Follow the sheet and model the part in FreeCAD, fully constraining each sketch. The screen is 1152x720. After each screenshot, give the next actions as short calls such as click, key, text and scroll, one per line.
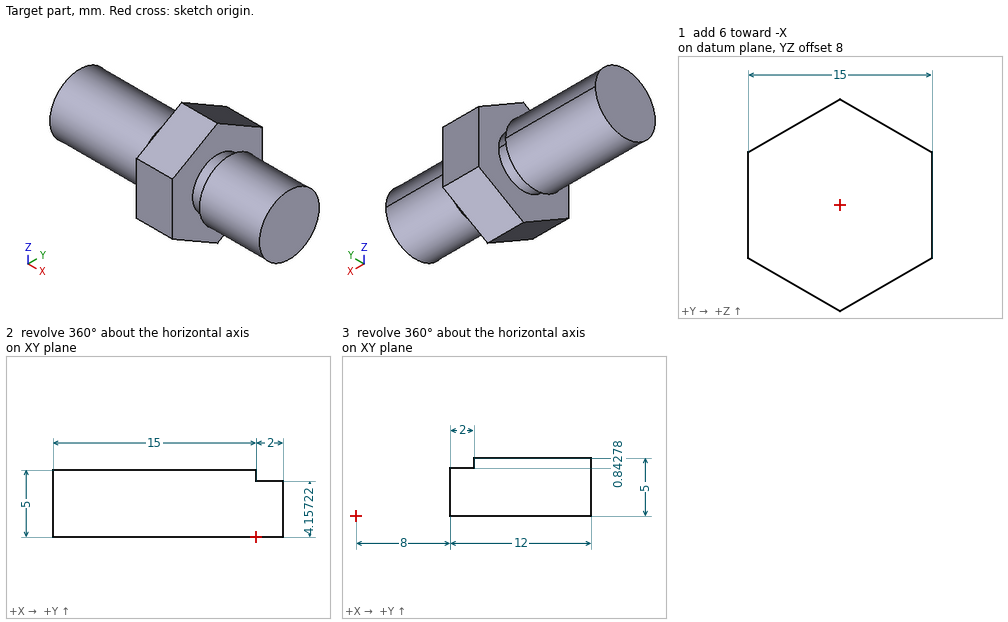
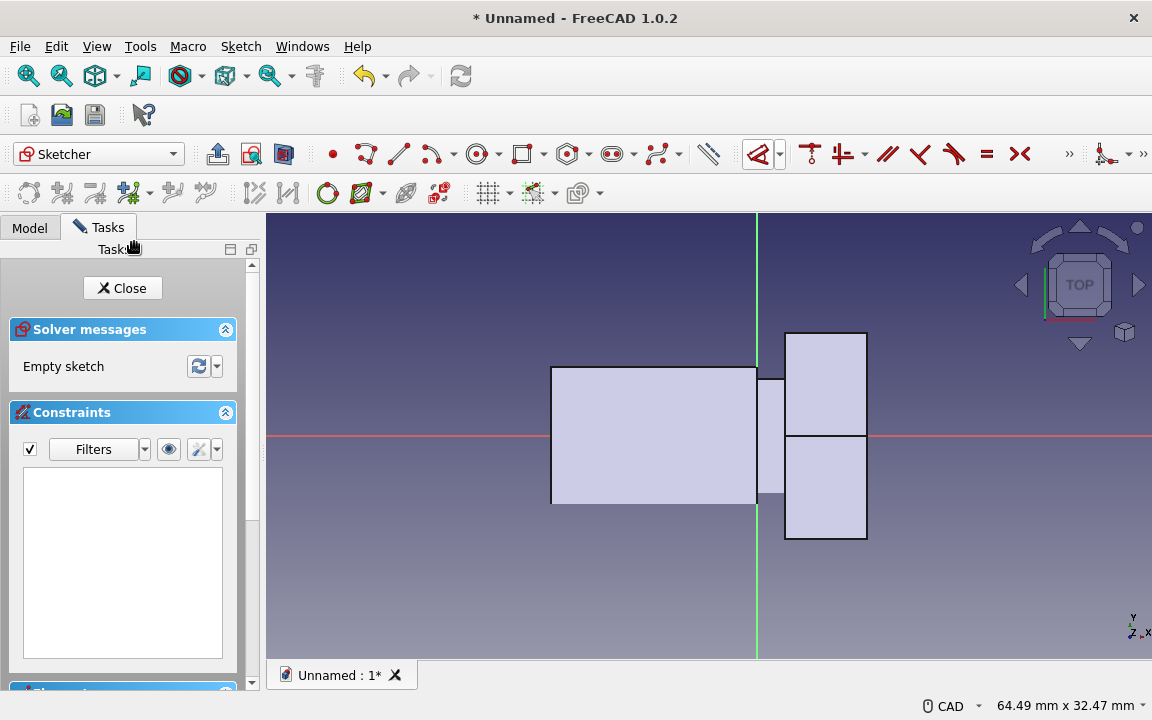
click(284, 154)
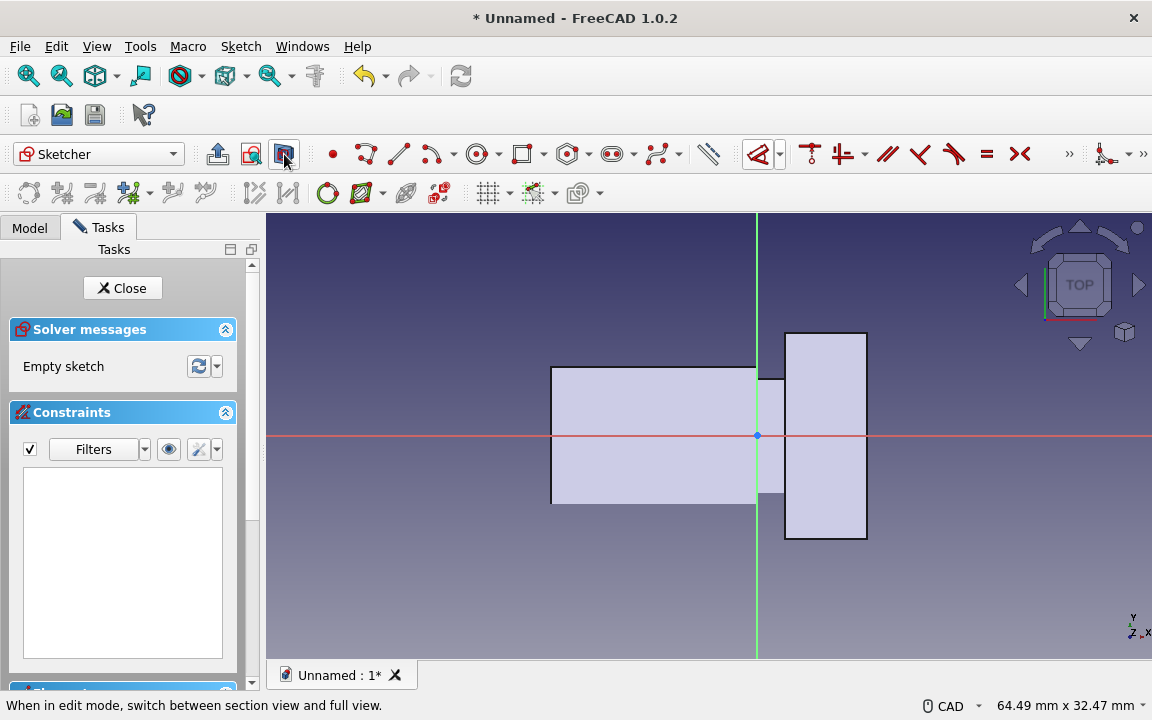
scroll(640, 436, down, 5)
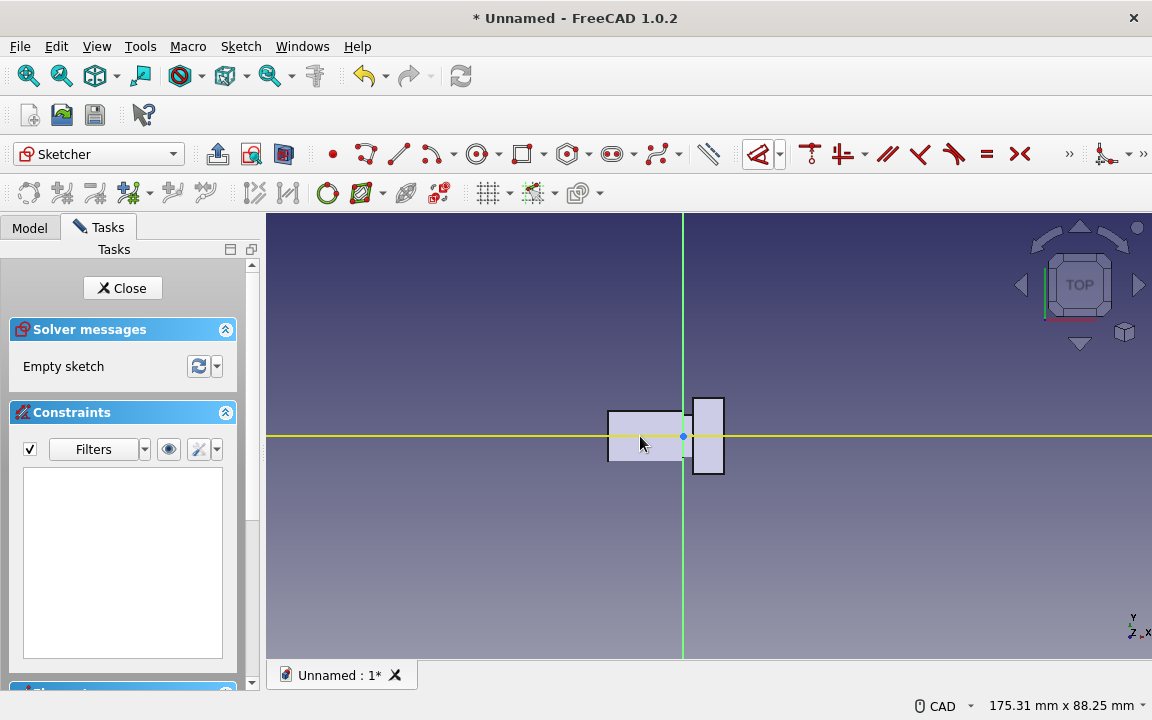
scroll(757, 421, up, 8)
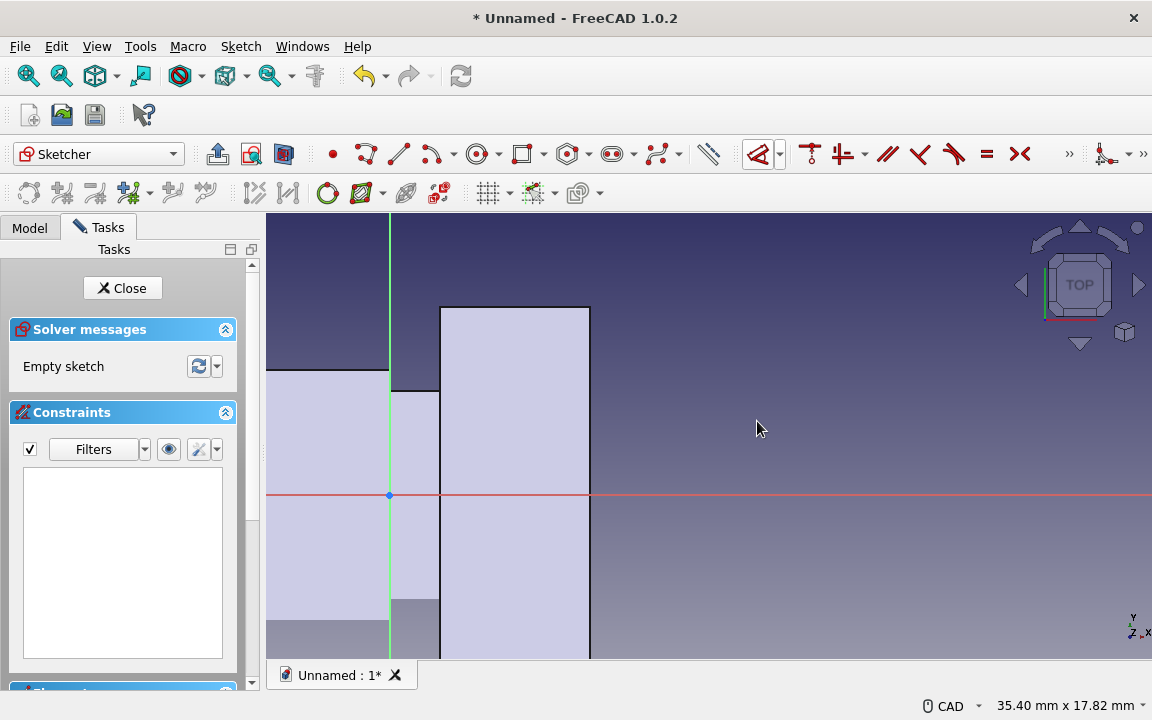
key(g)
key(m)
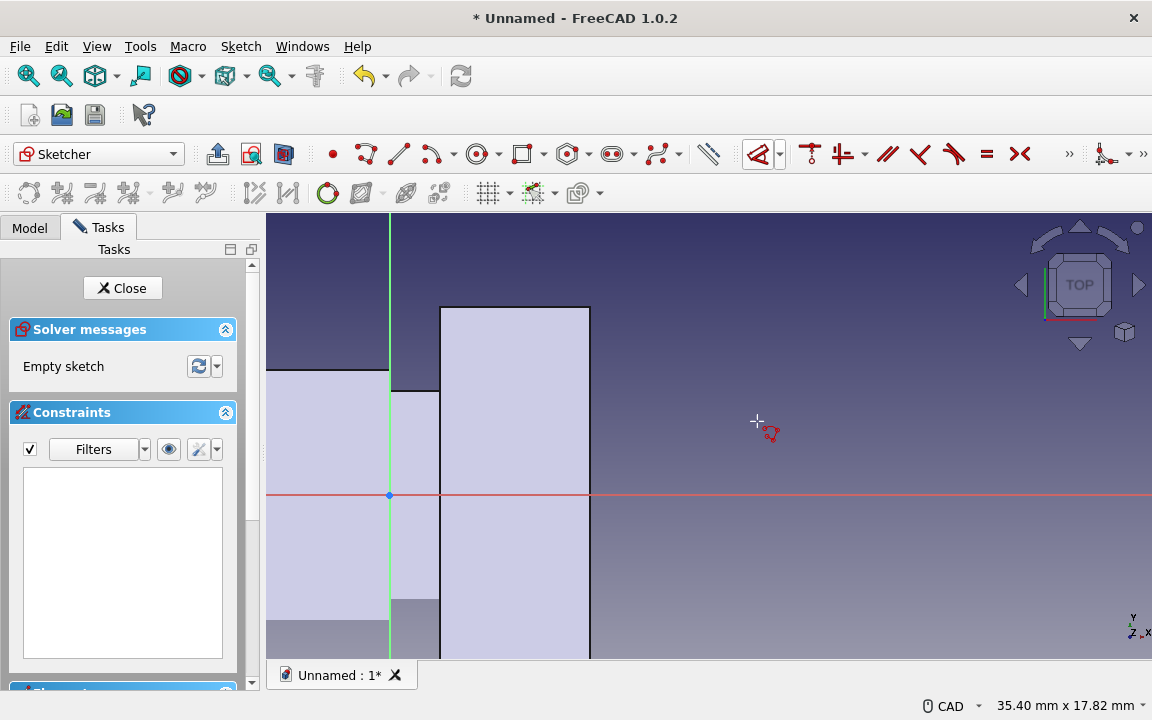
click(590, 495)
click(891, 486)
click(891, 370)
click(640, 370)
click(640, 391)
click(590, 391)
click(590, 495)
key(Escape)
key(Escape)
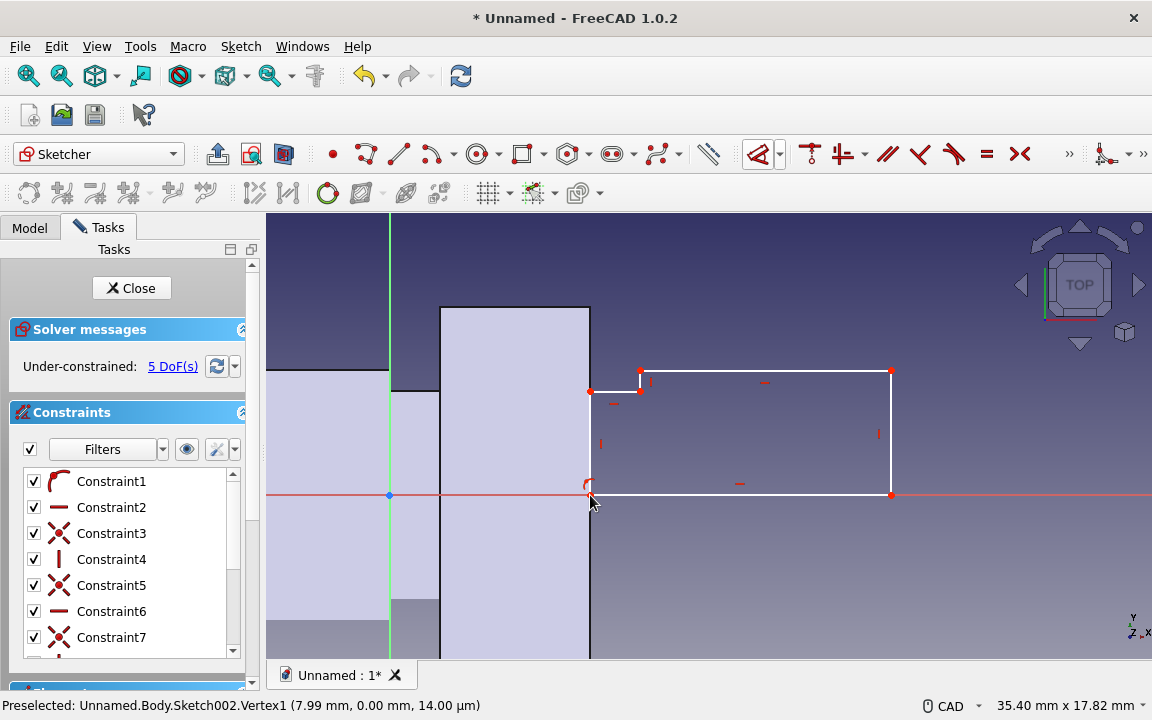
click(891, 458)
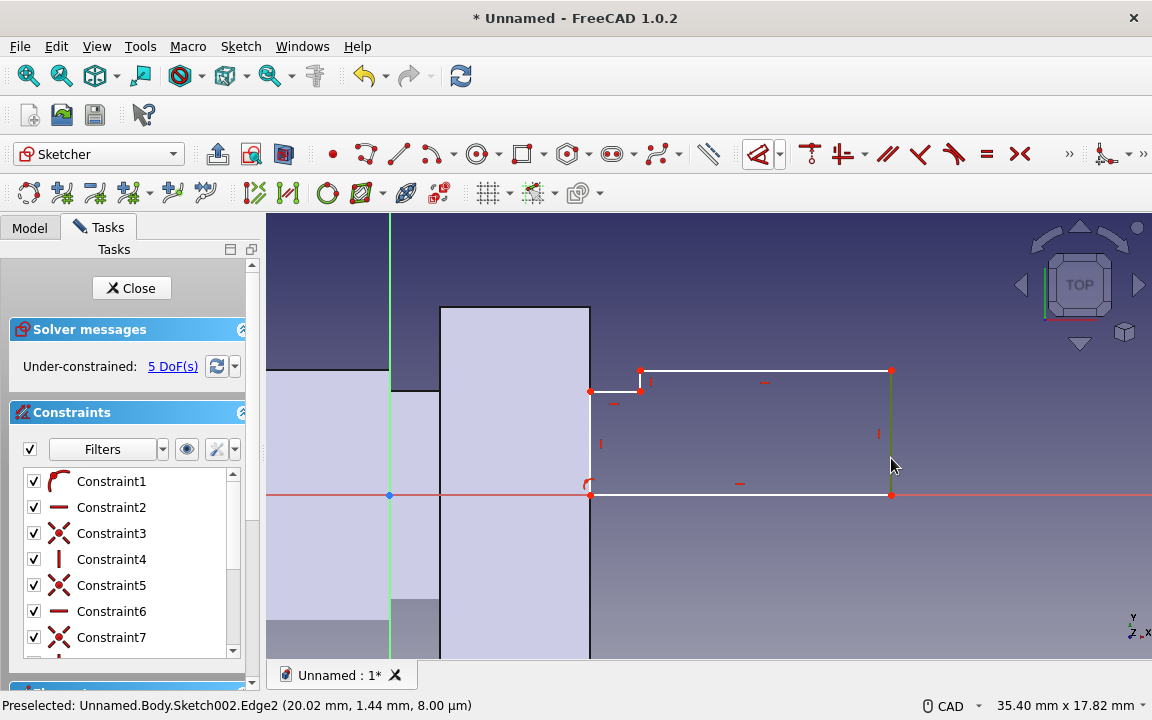
click(780, 154)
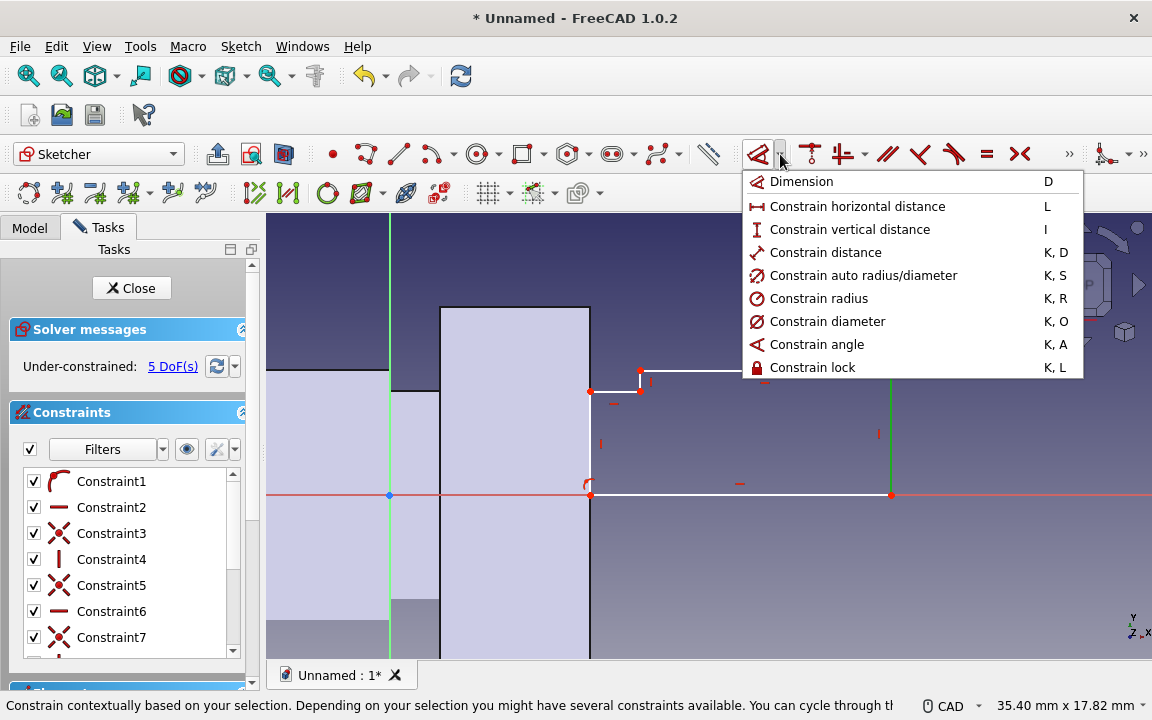
click(913, 230)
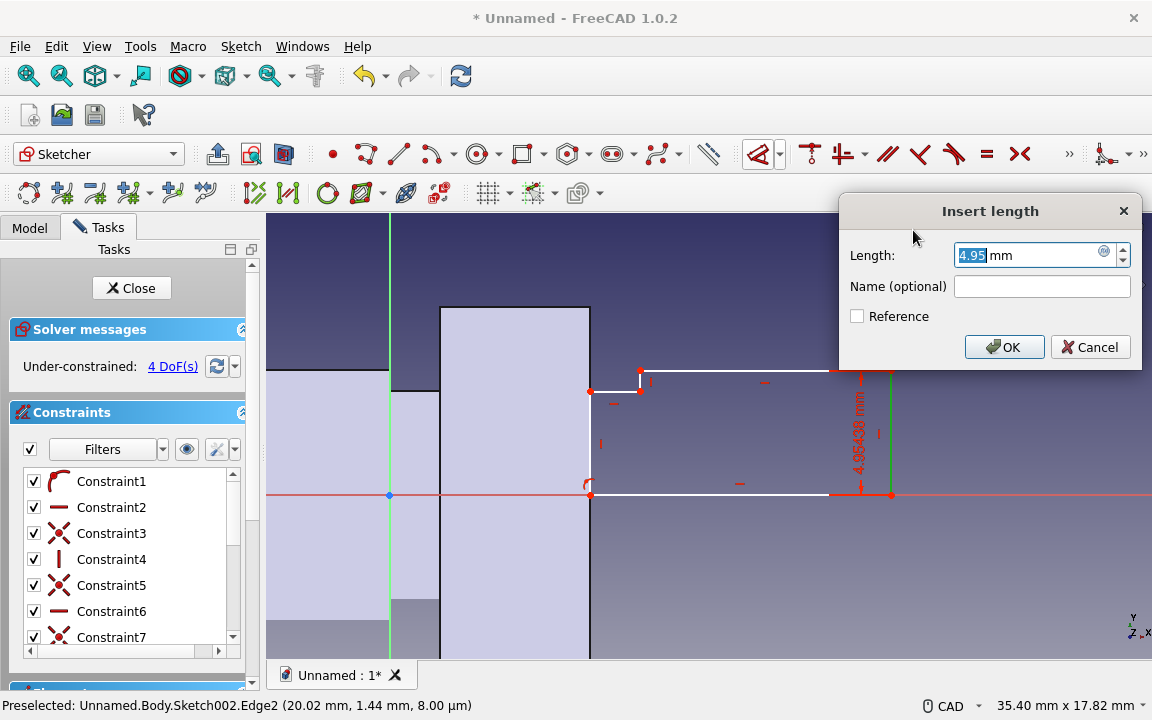
text(5)
key(Return)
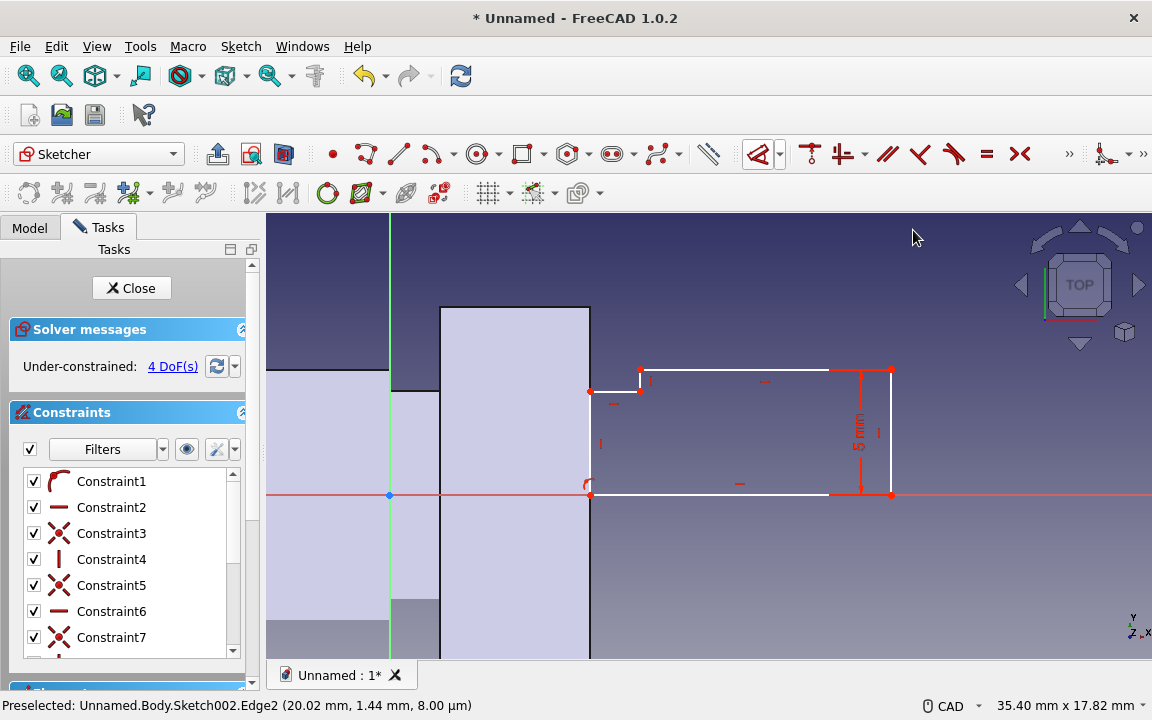
click(625, 392)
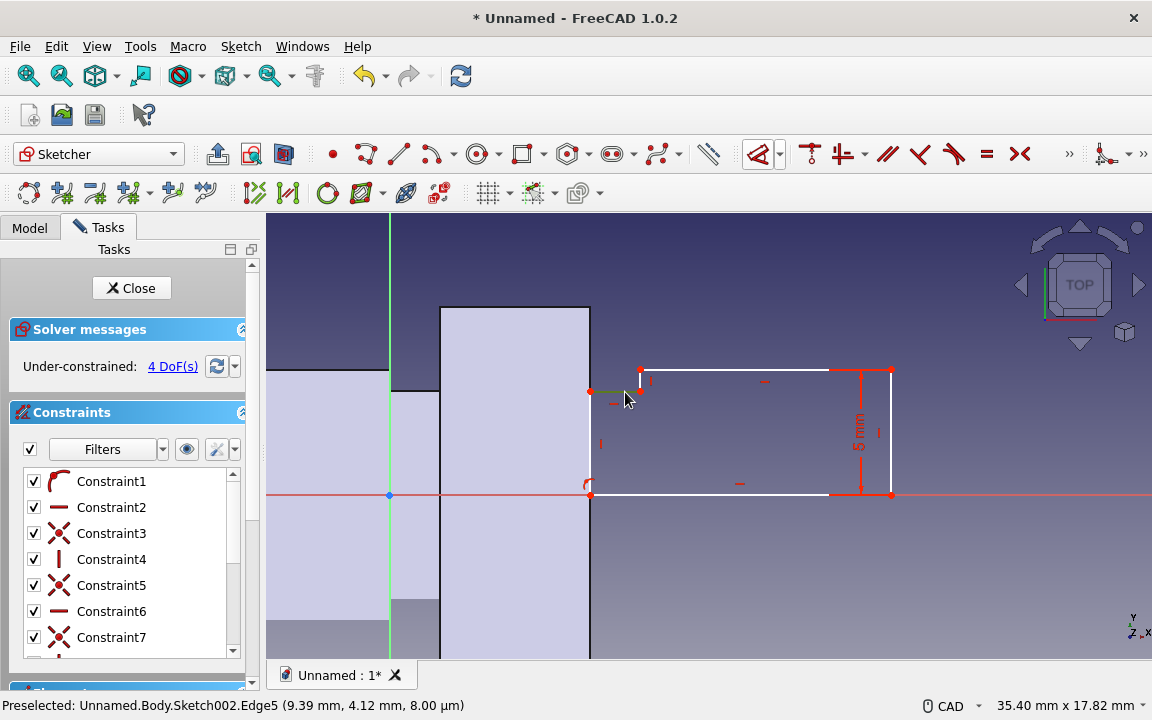
key(l)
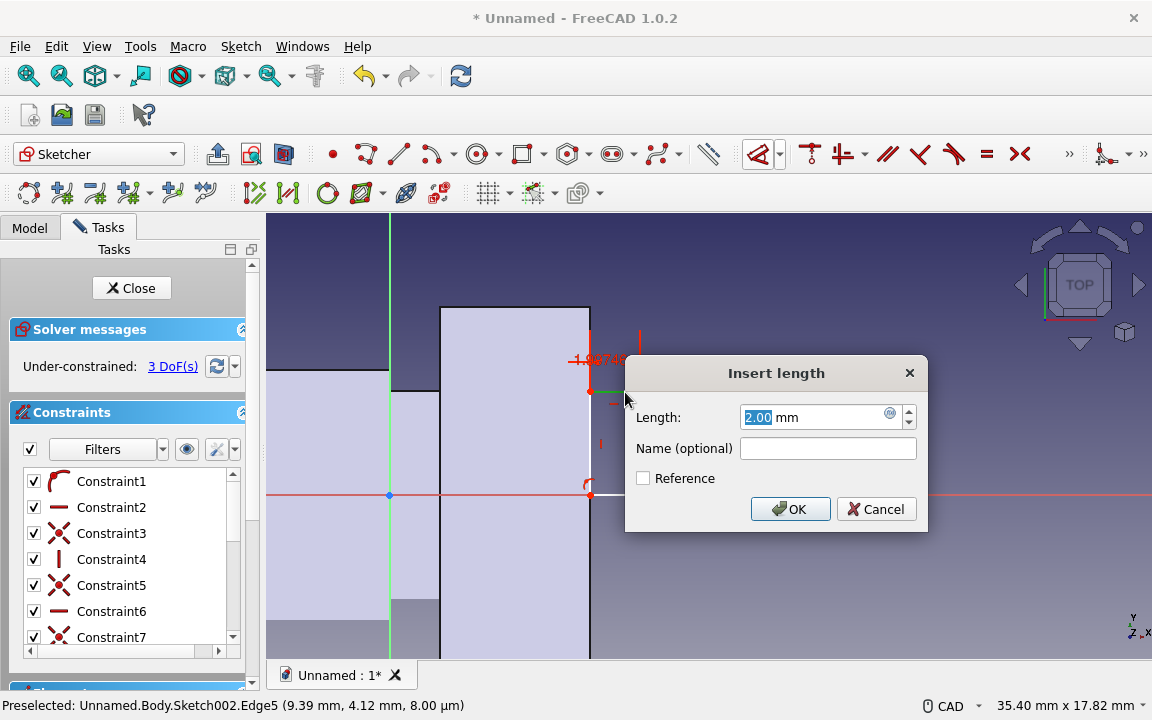
text(2)
key(Return)